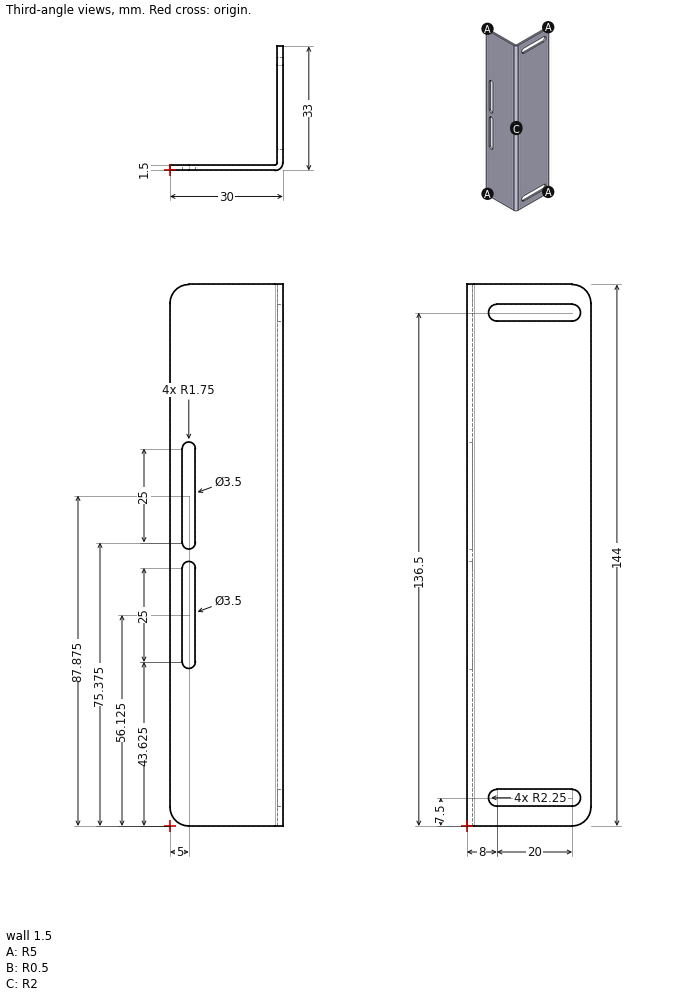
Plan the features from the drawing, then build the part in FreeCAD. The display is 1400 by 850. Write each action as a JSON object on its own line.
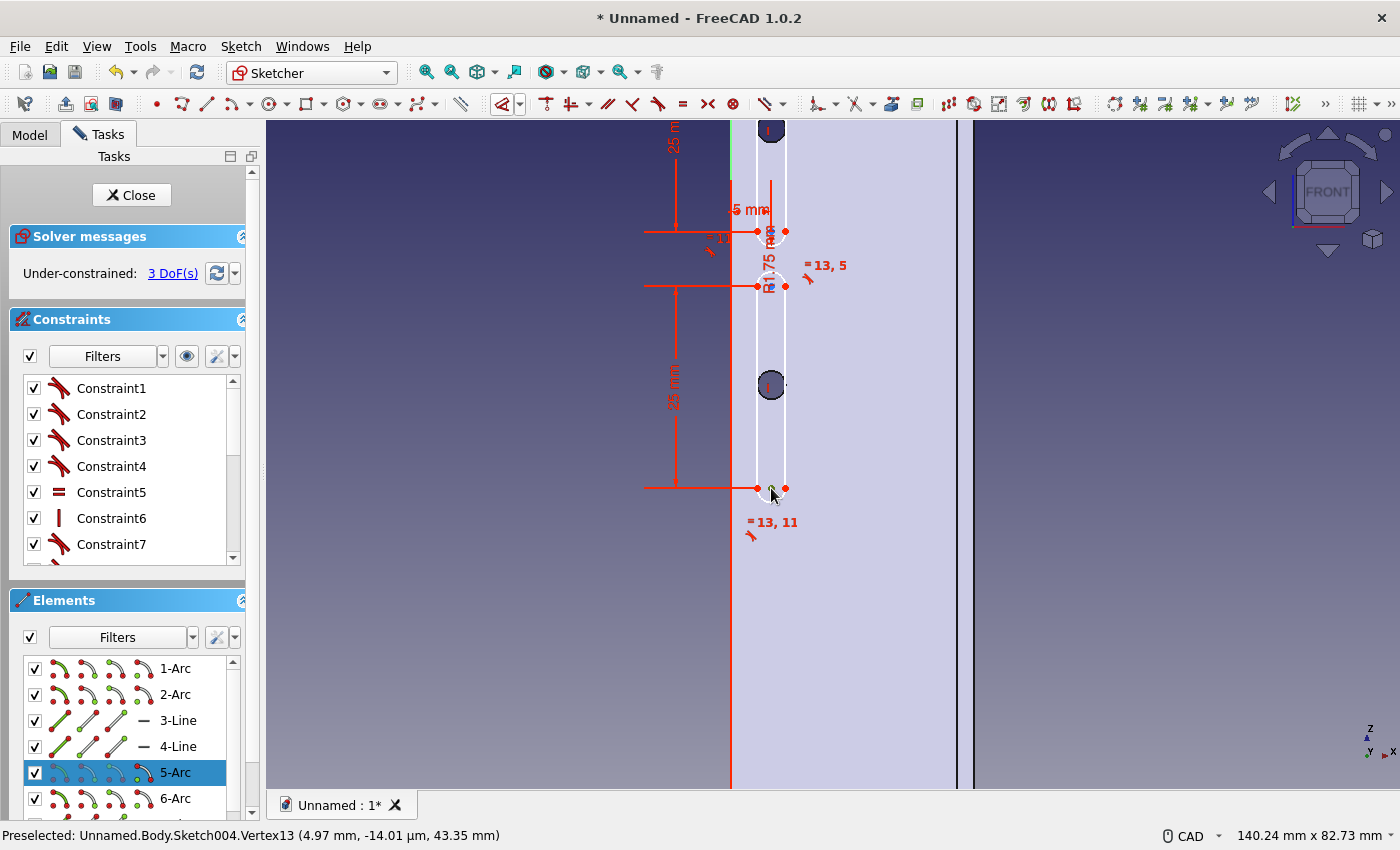
{"action": "left_click", "coordinate": [520, 104]}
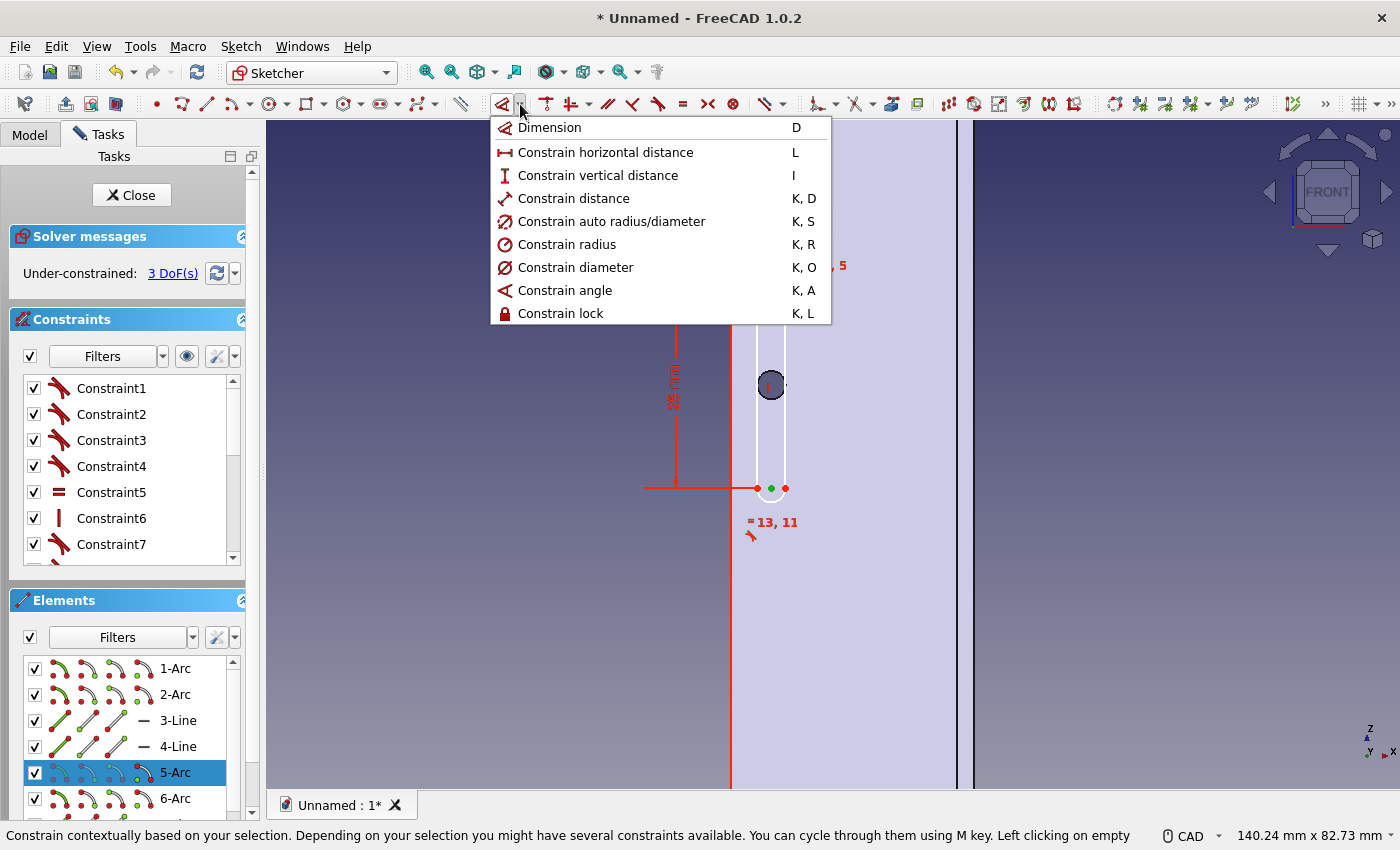
{"action": "left_click", "coordinate": [661, 152]}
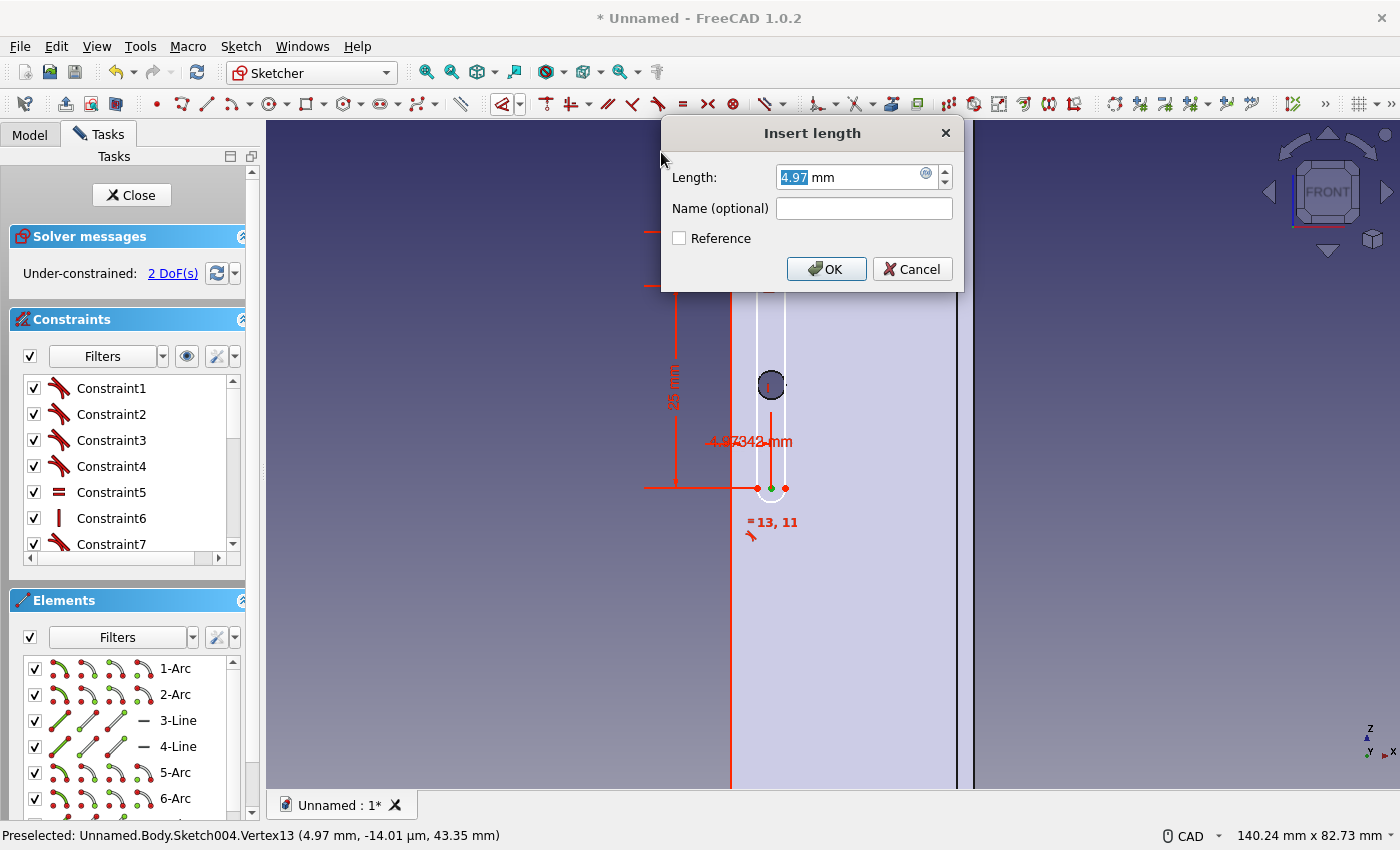
{"action": "type", "text": "5"}
{"action": "key", "text": "Return"}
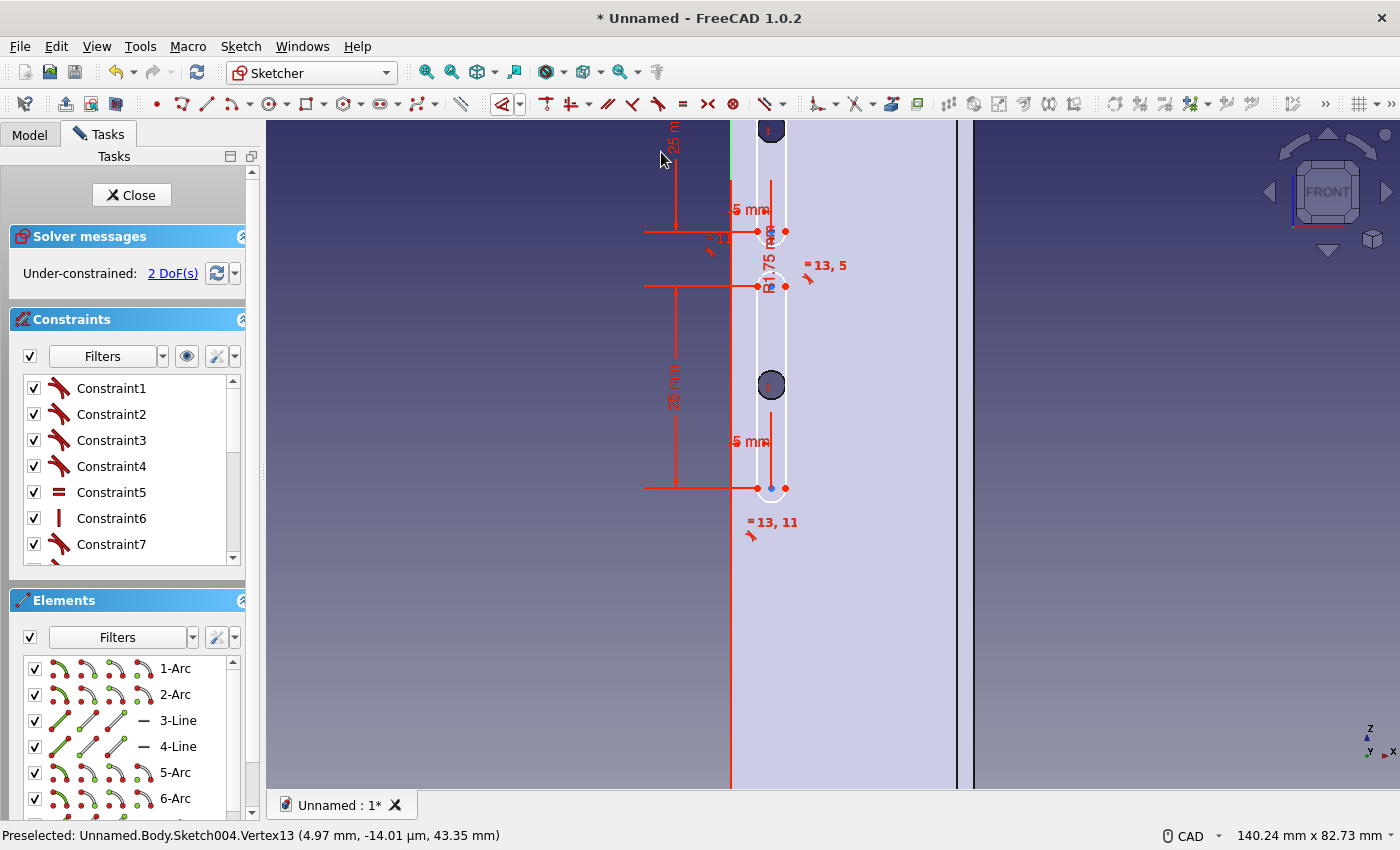
{"action": "left_click", "coordinate": [757, 232]}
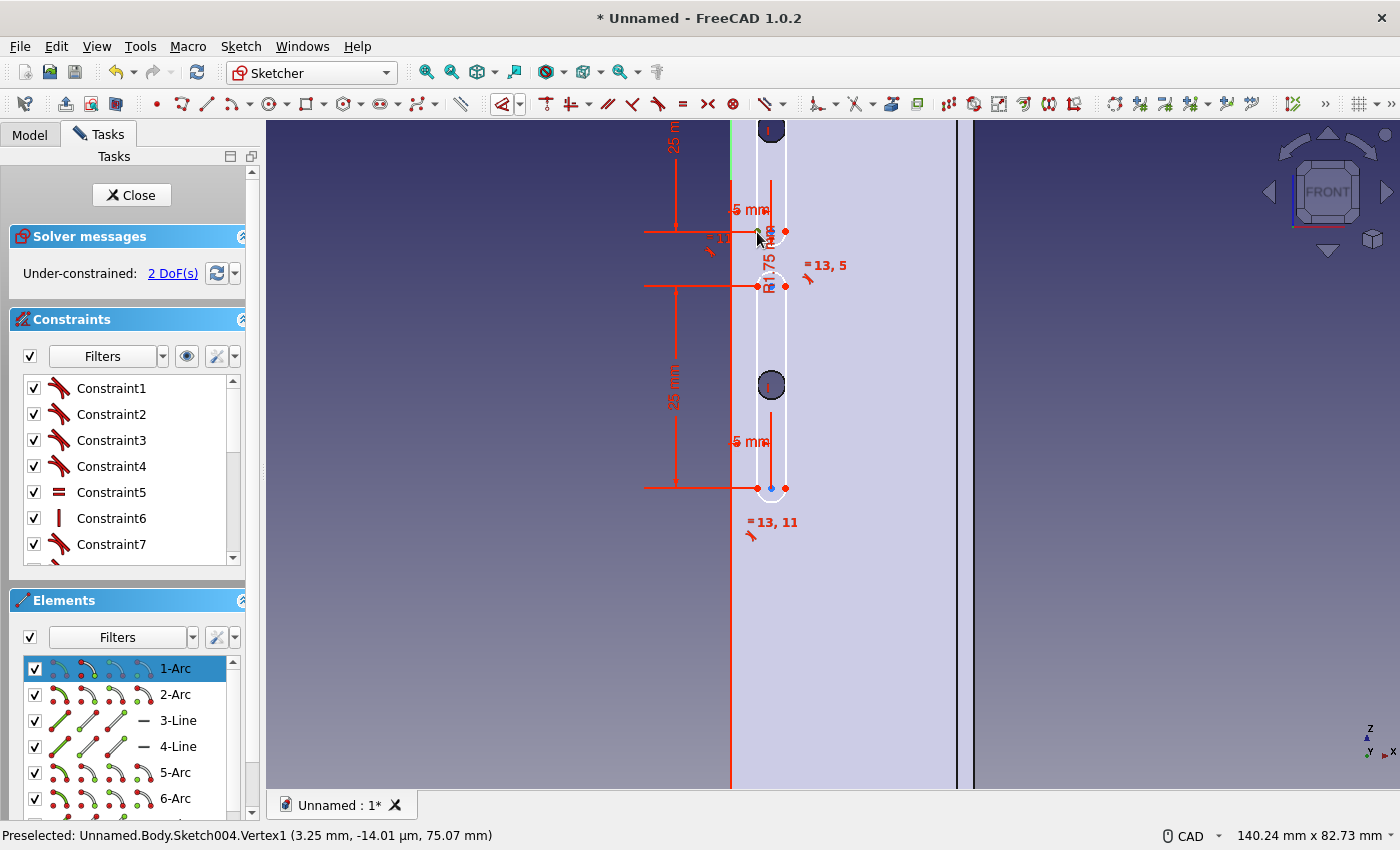
{"action": "left_click", "coordinate": [520, 104]}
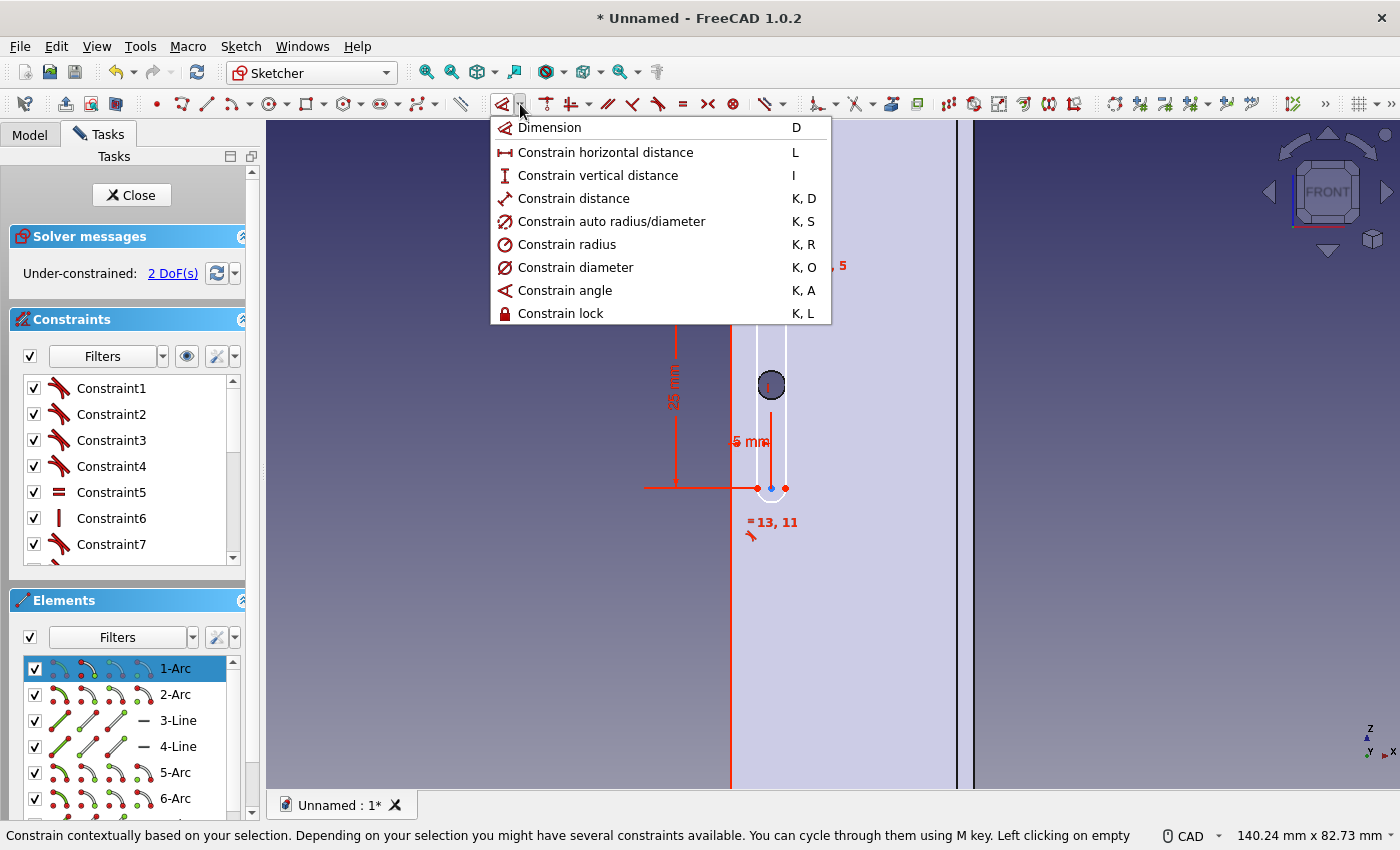
{"action": "left_click", "coordinate": [661, 176]}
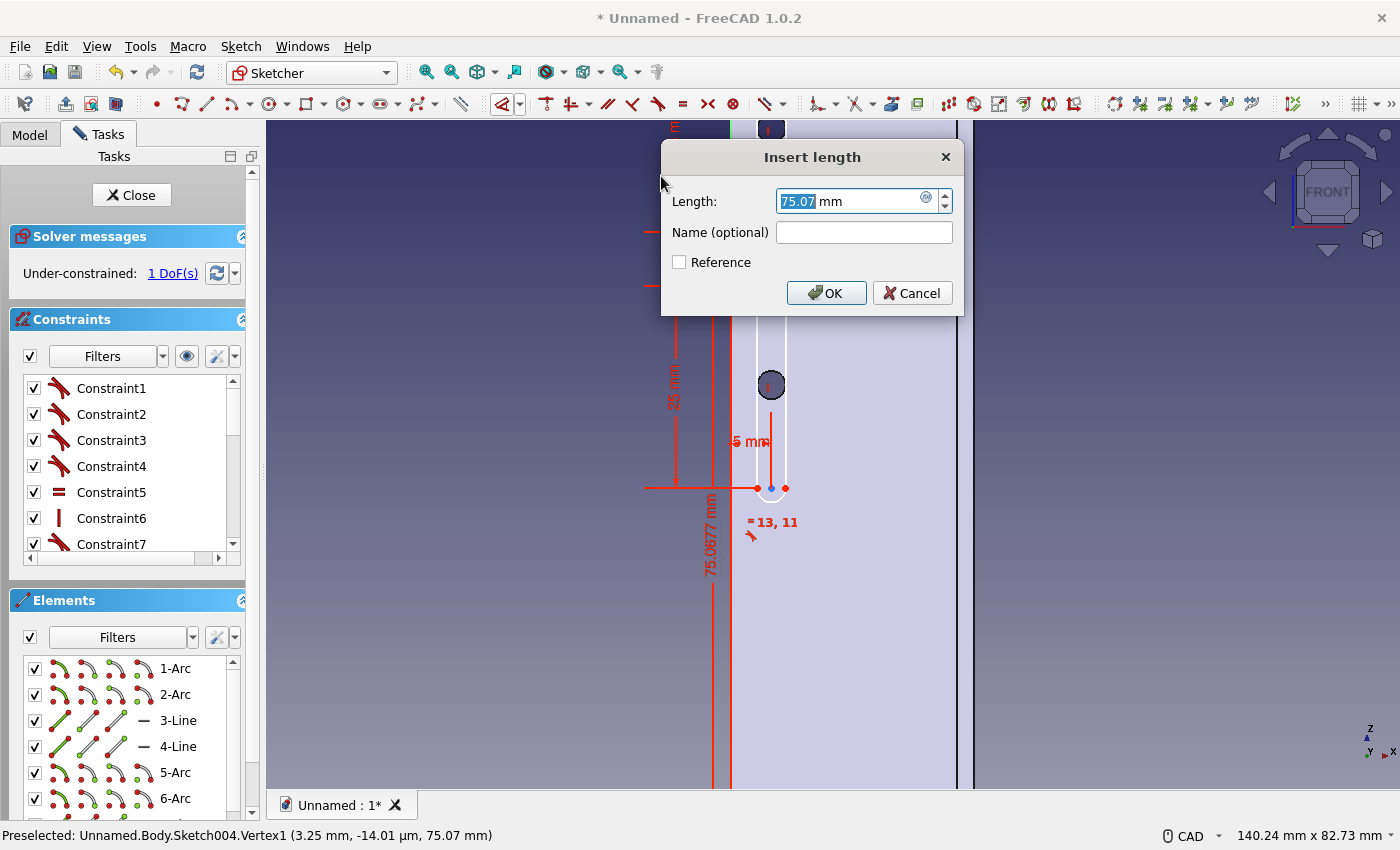
{"action": "type", "text": "75.375"}
{"action": "key", "text": "Return"}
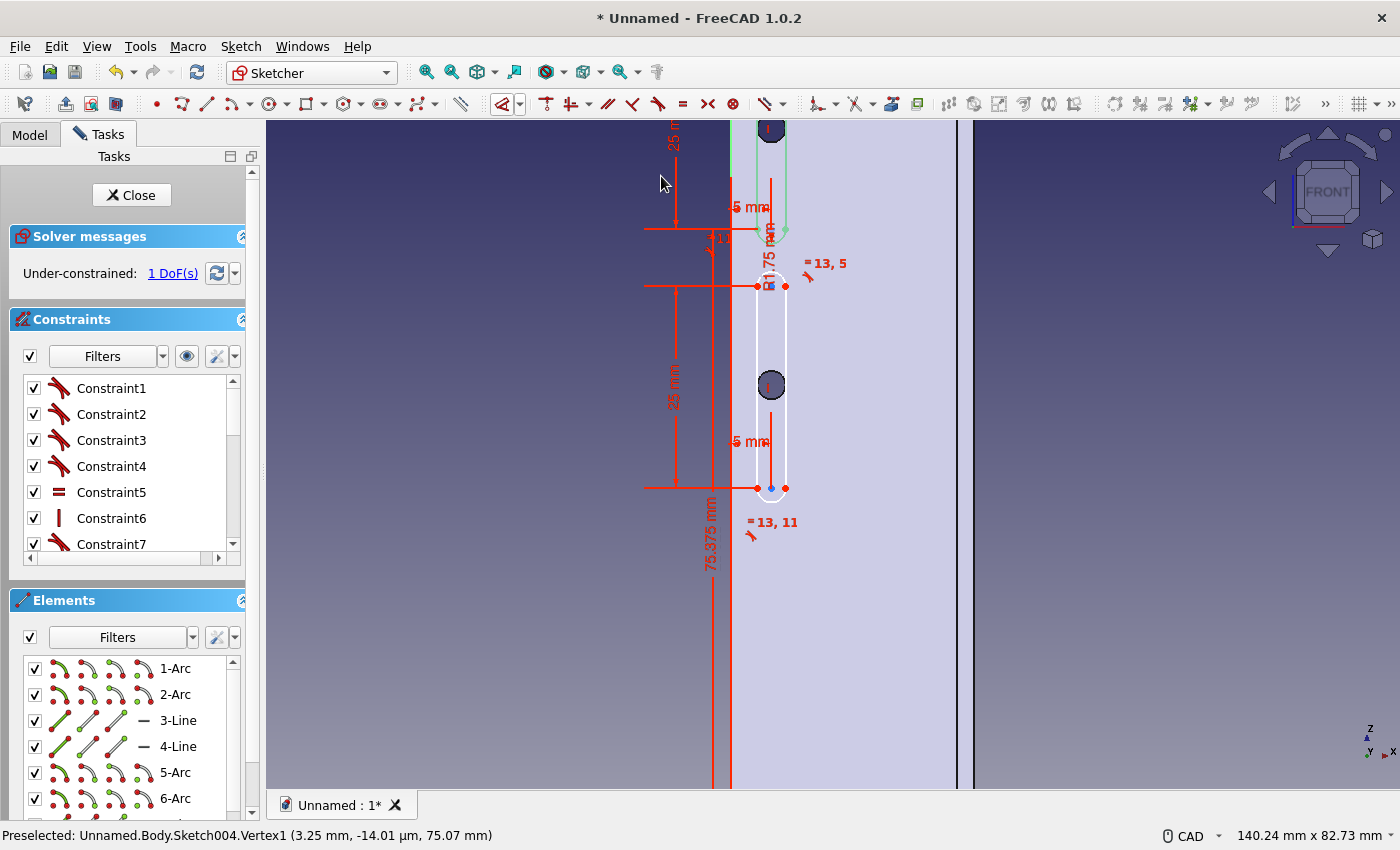
{"action": "left_click", "coordinate": [757, 488]}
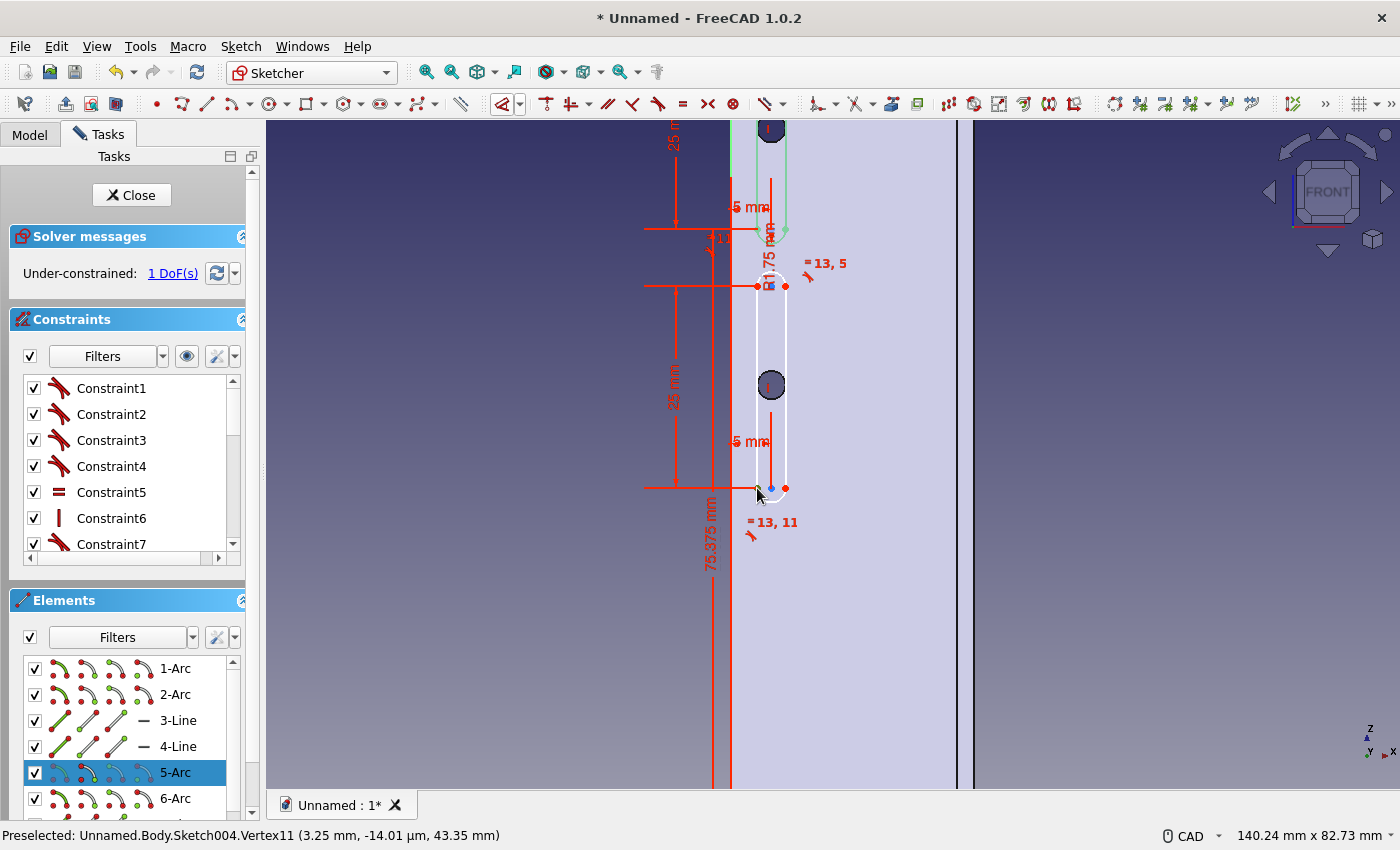
{"action": "key", "text": "i"}